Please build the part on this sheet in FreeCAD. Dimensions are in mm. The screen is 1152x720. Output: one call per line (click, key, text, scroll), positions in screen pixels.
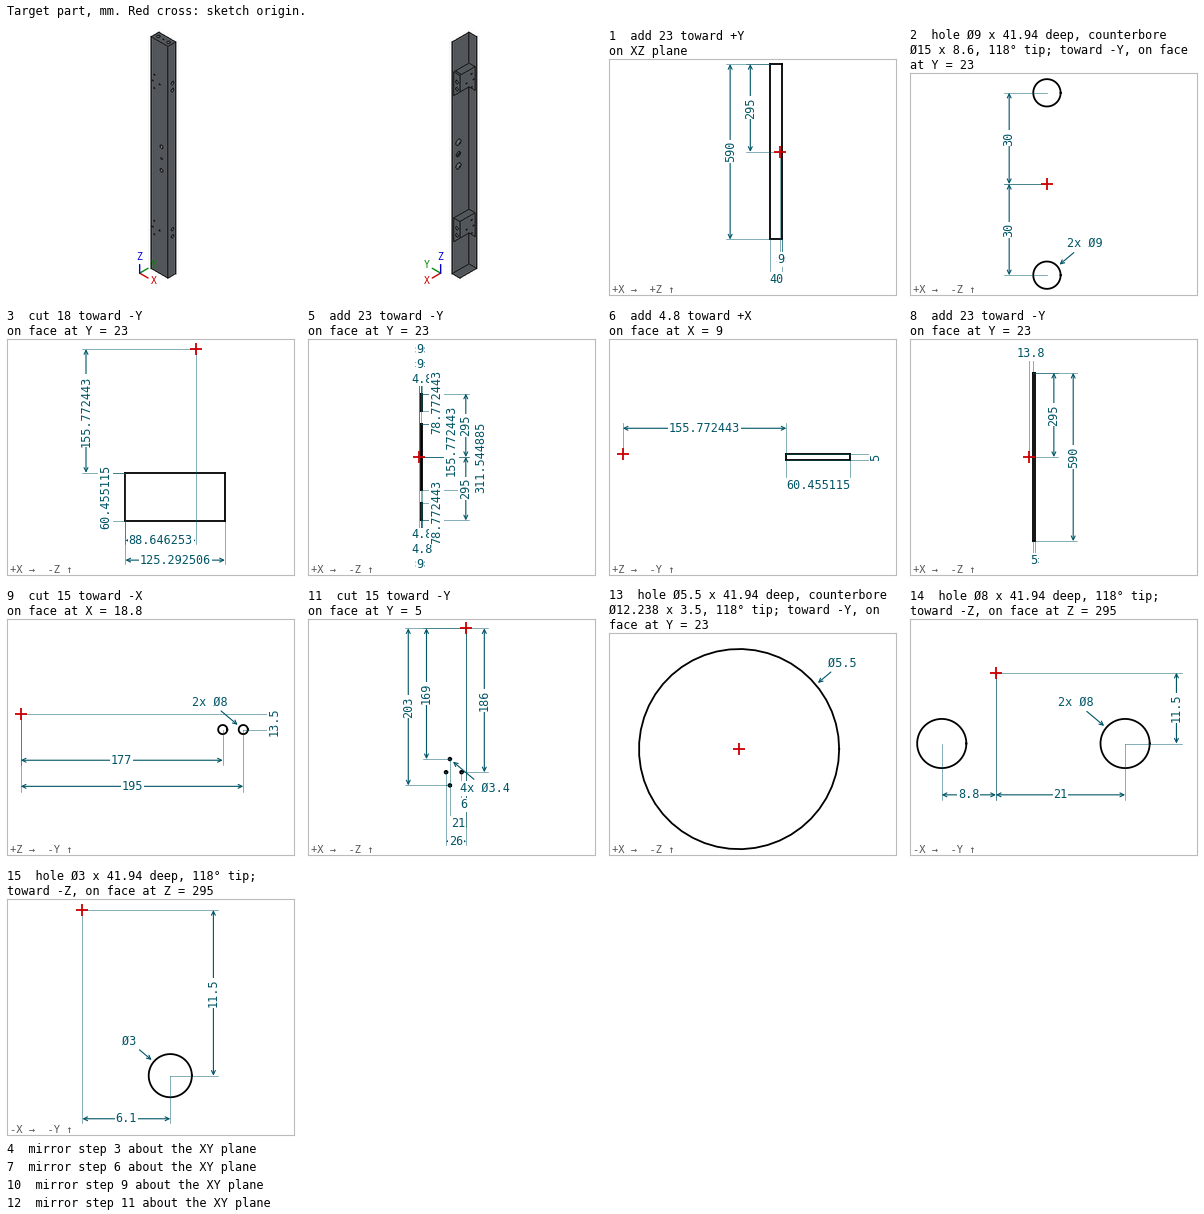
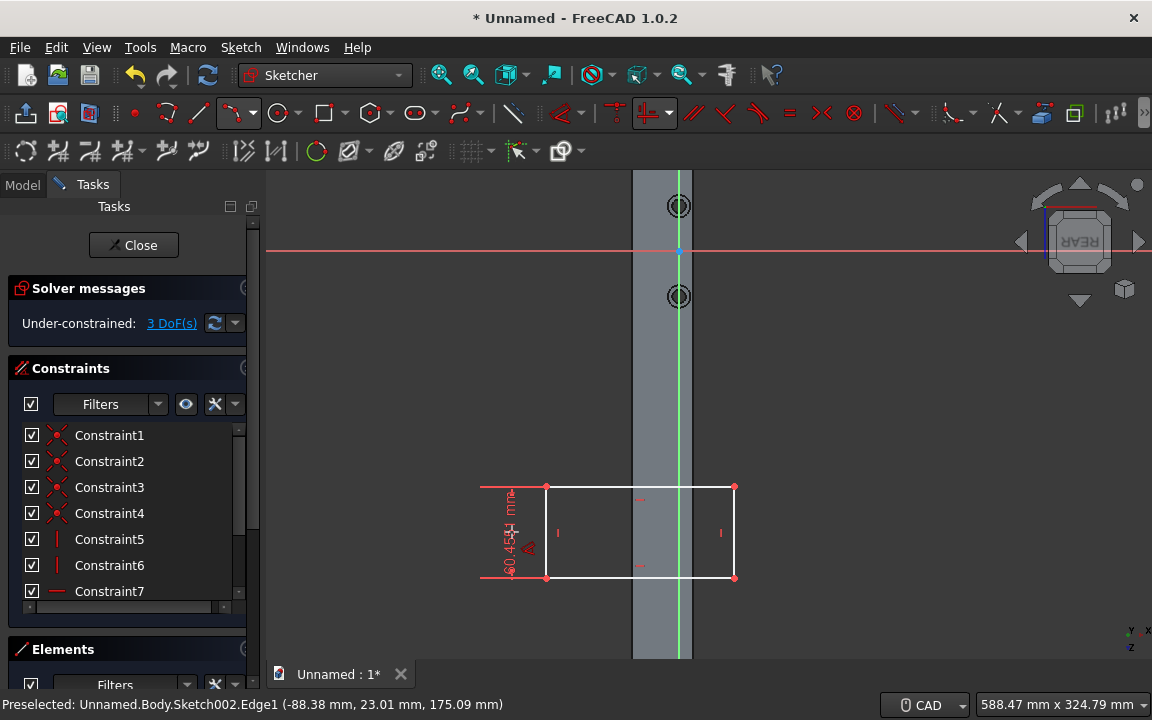
click(602, 578)
click(640, 612)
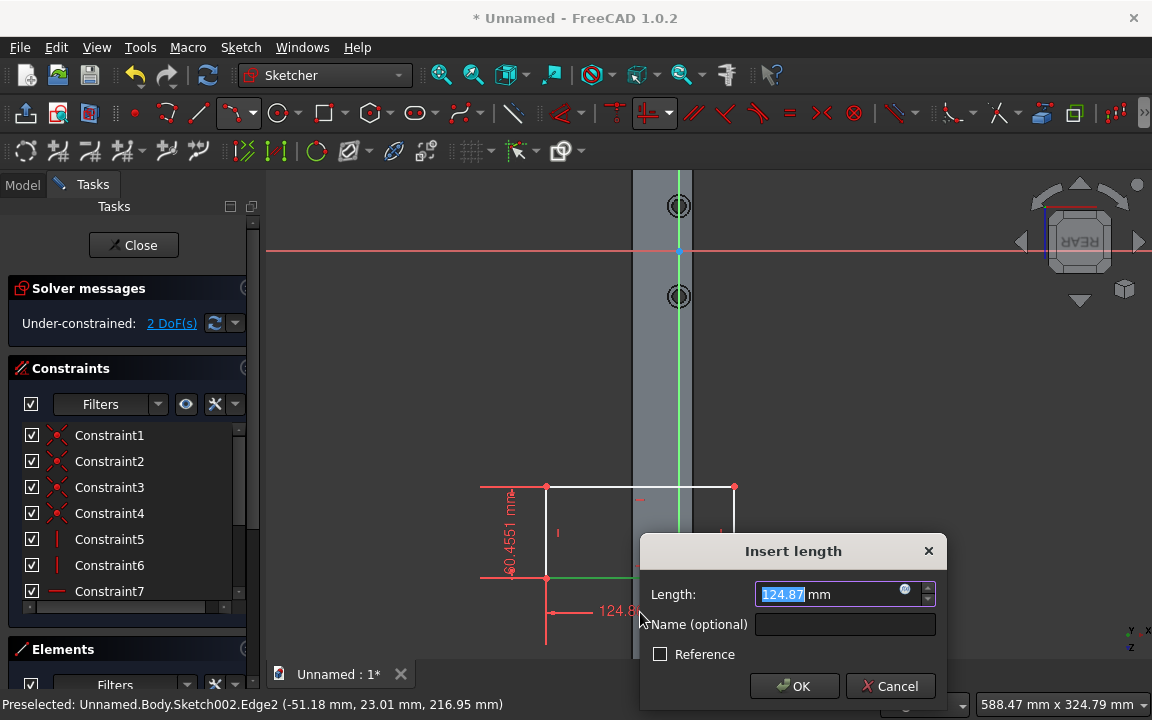
text(125.292506)
key(Return)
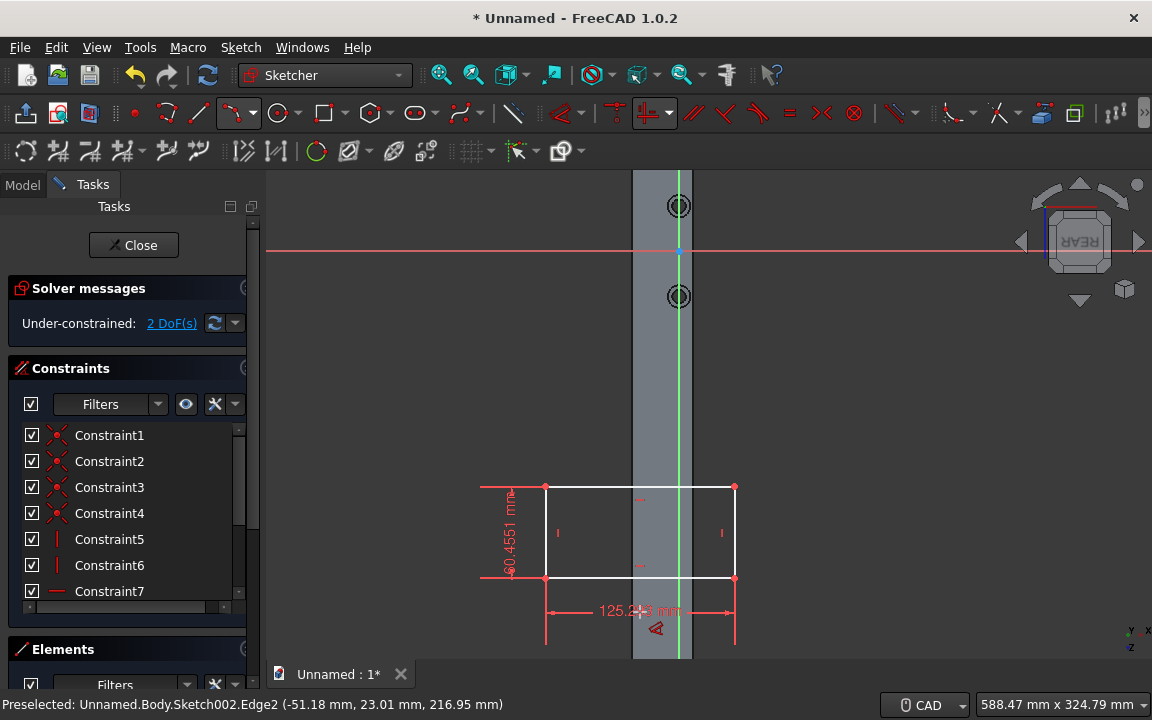
click(546, 487)
click(612, 217)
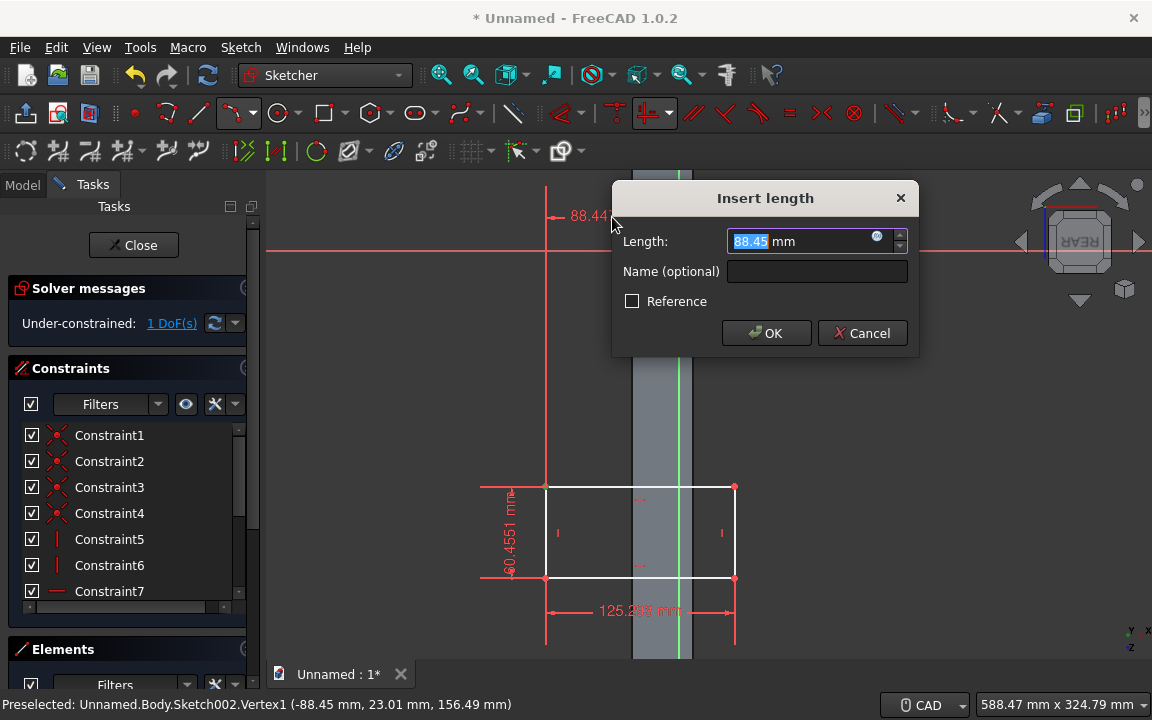
text(88.646253)
key(Return)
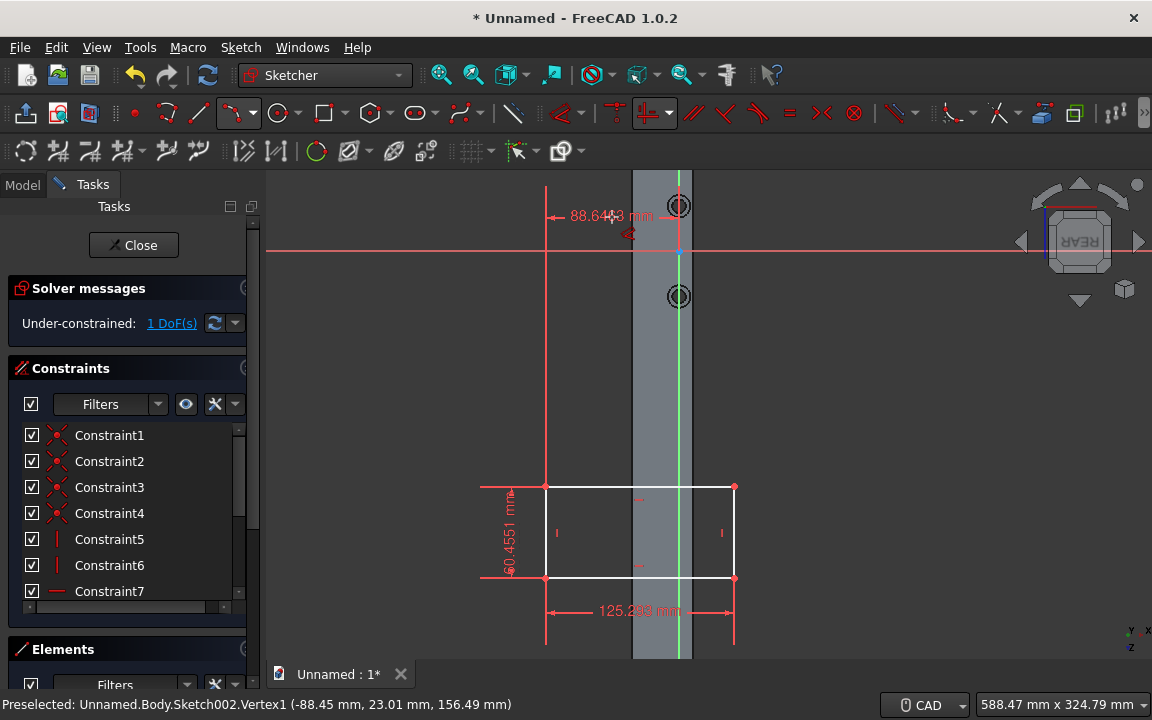
click(546, 487)
click(512, 369)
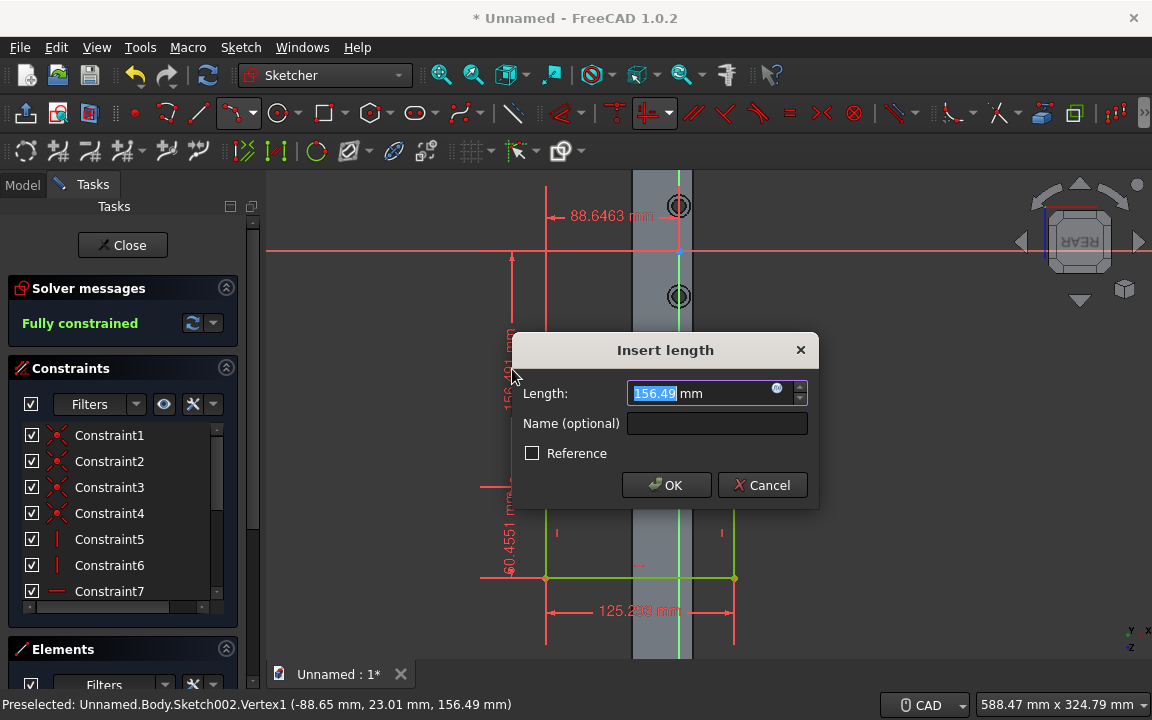
text(155.772443)
key(Return)
key(Escape)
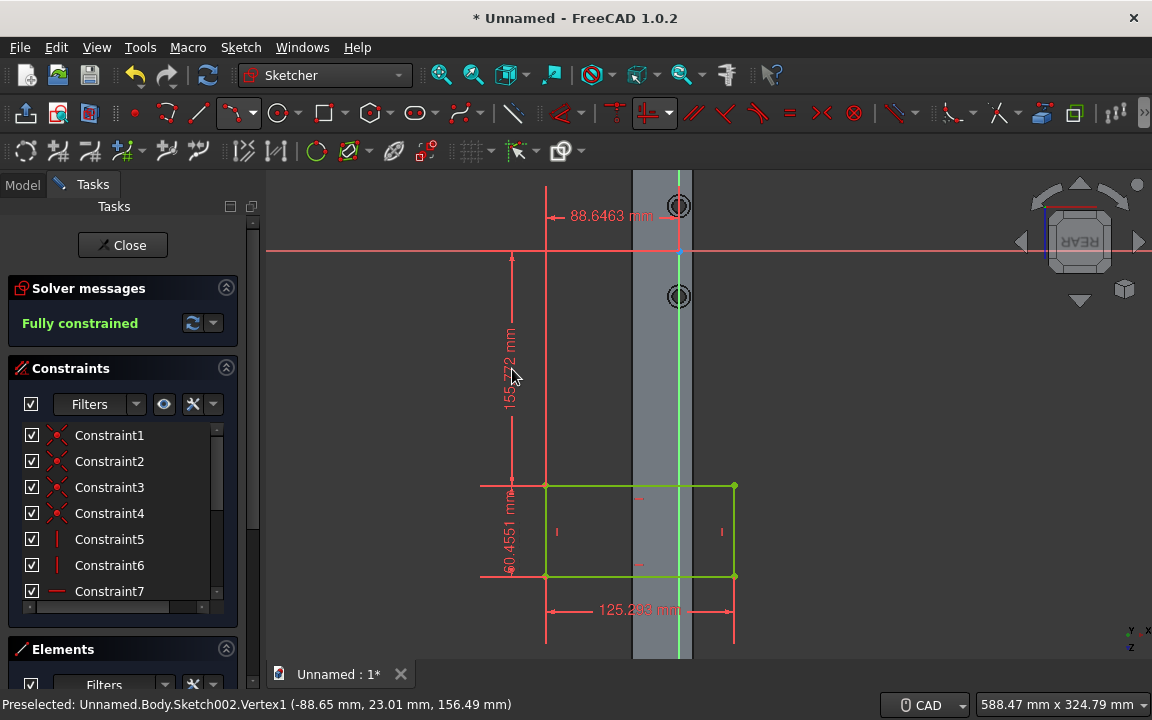
click(123, 245)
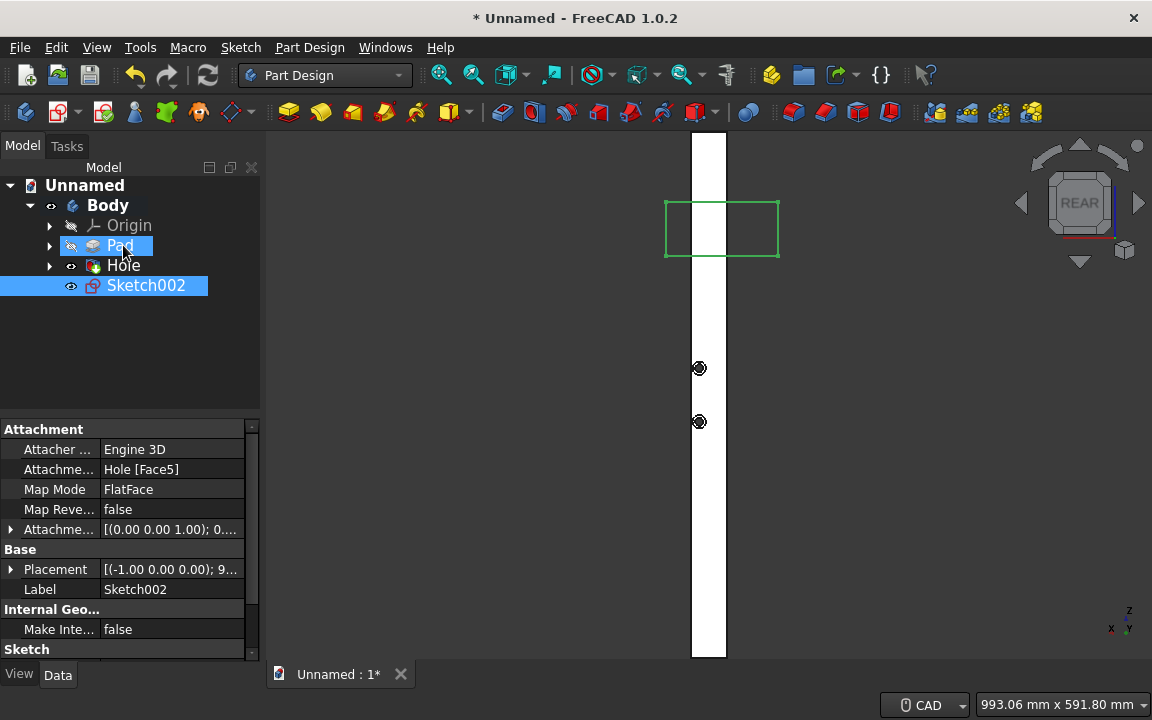
click(504, 112)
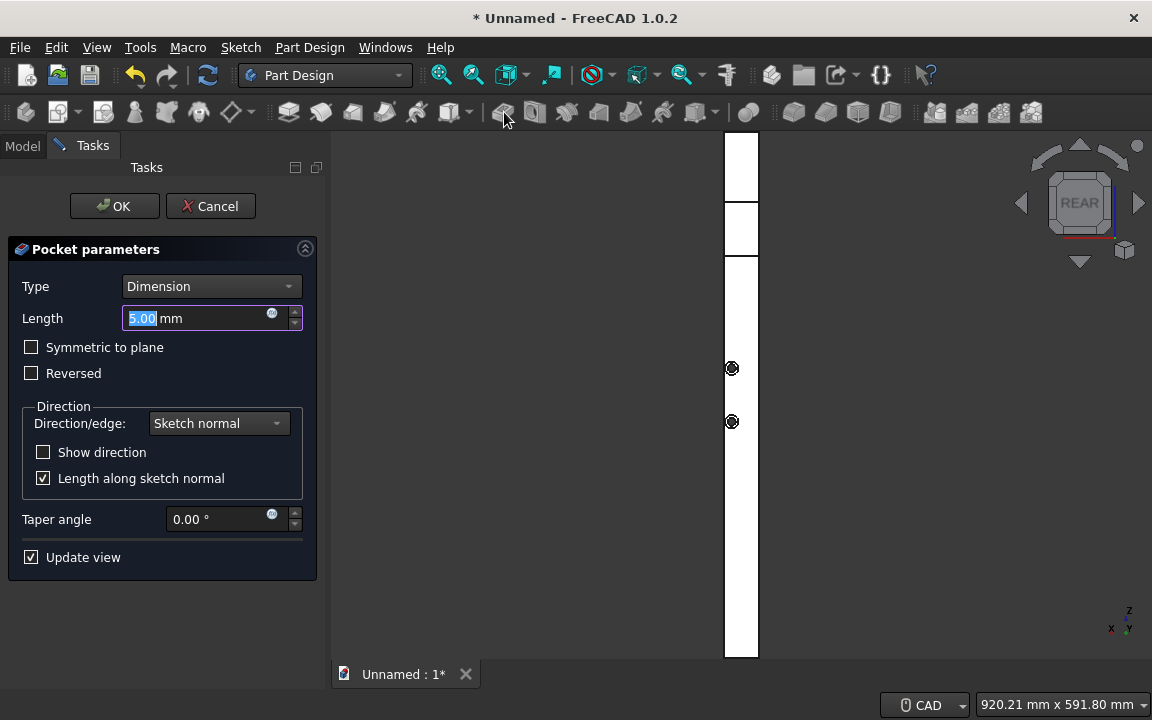
text(18)
key(Tab)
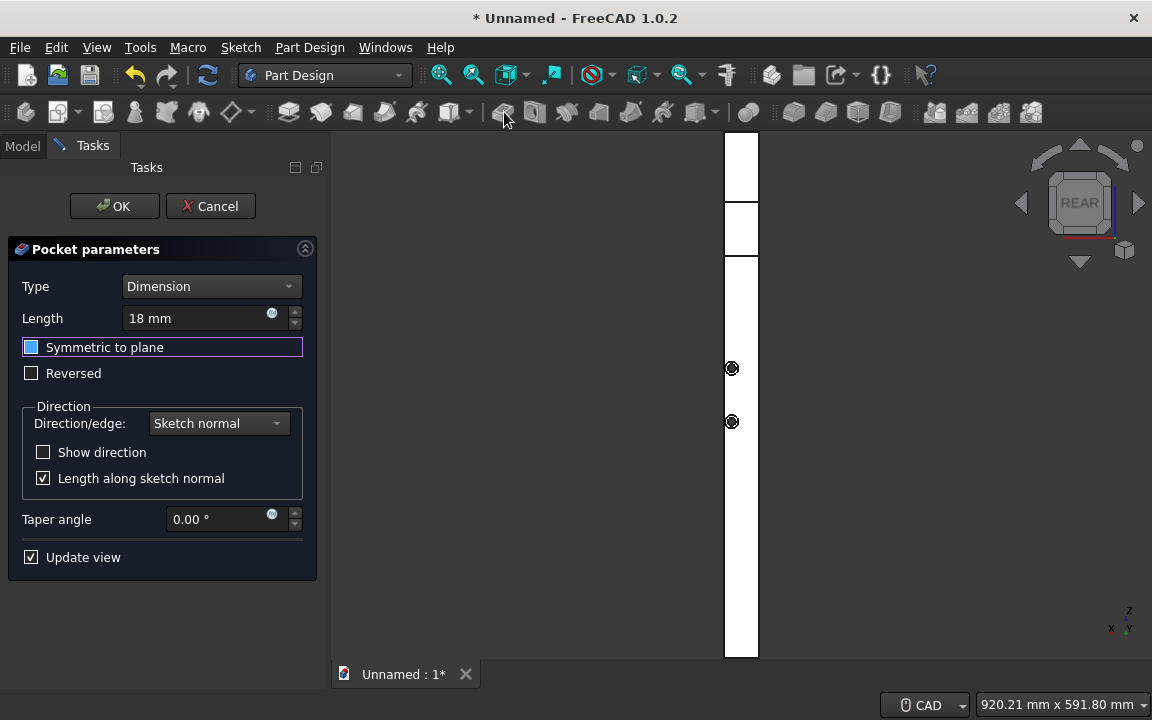
click(115, 206)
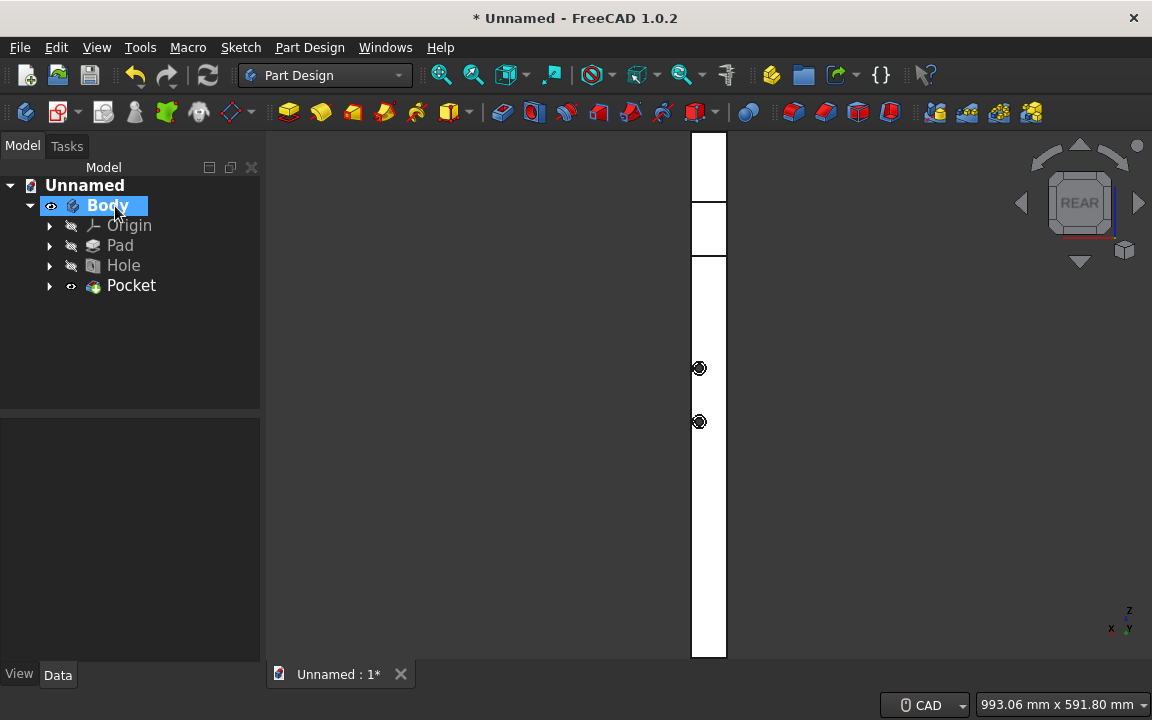
click(116, 286)